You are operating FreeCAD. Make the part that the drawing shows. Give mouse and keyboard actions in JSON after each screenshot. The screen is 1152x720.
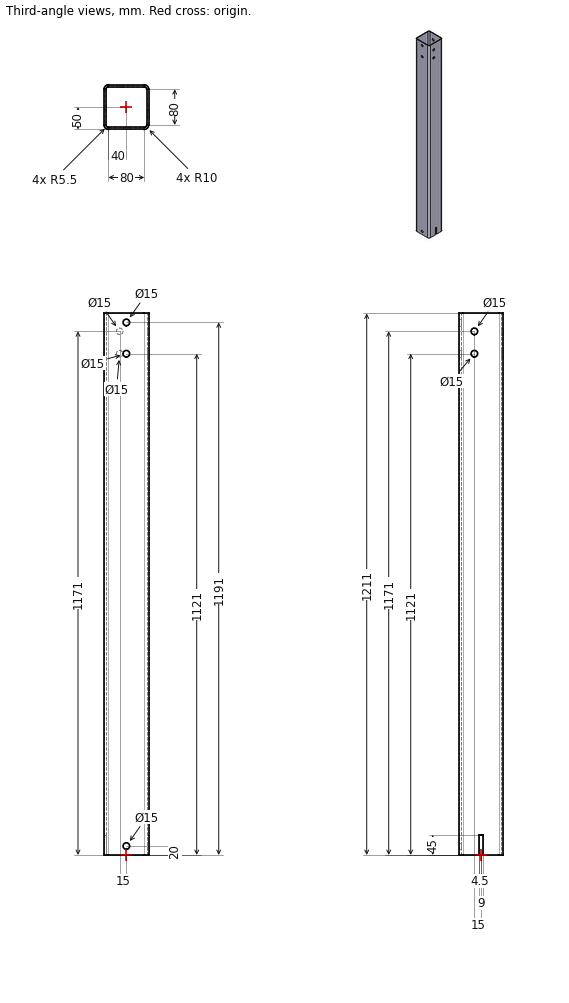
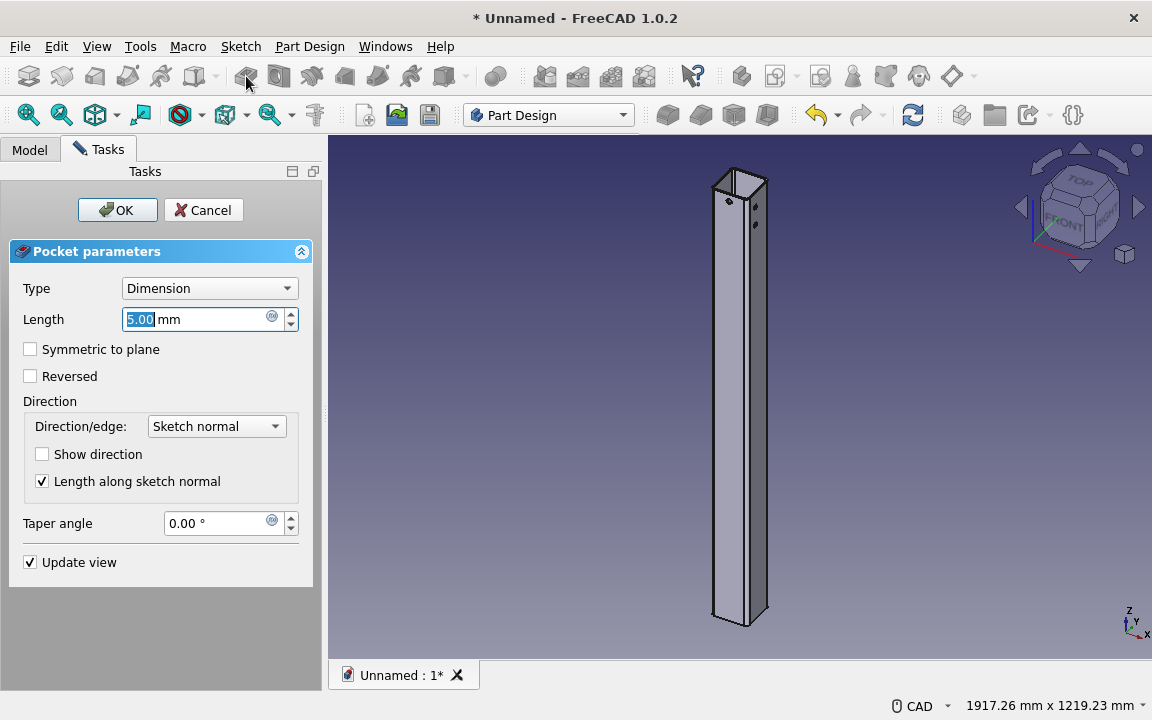
{"action": "left_click", "coordinate": [210, 288]}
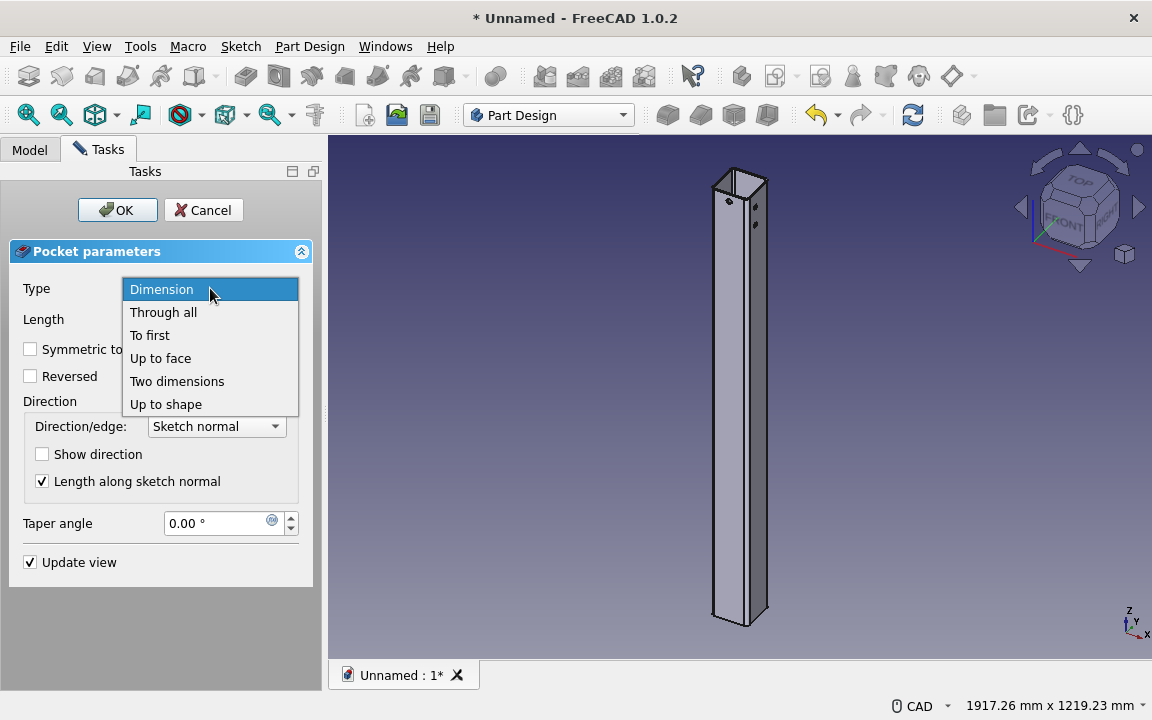
{"action": "left_click", "coordinate": [208, 336]}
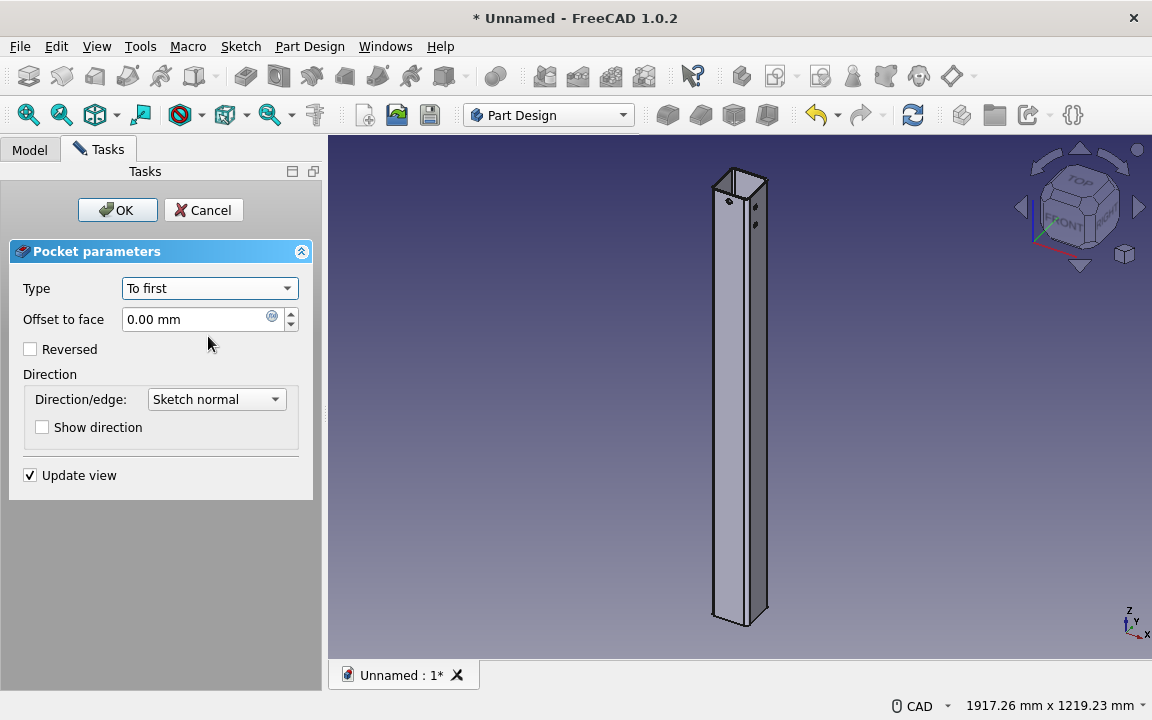
{"action": "left_click", "coordinate": [118, 210]}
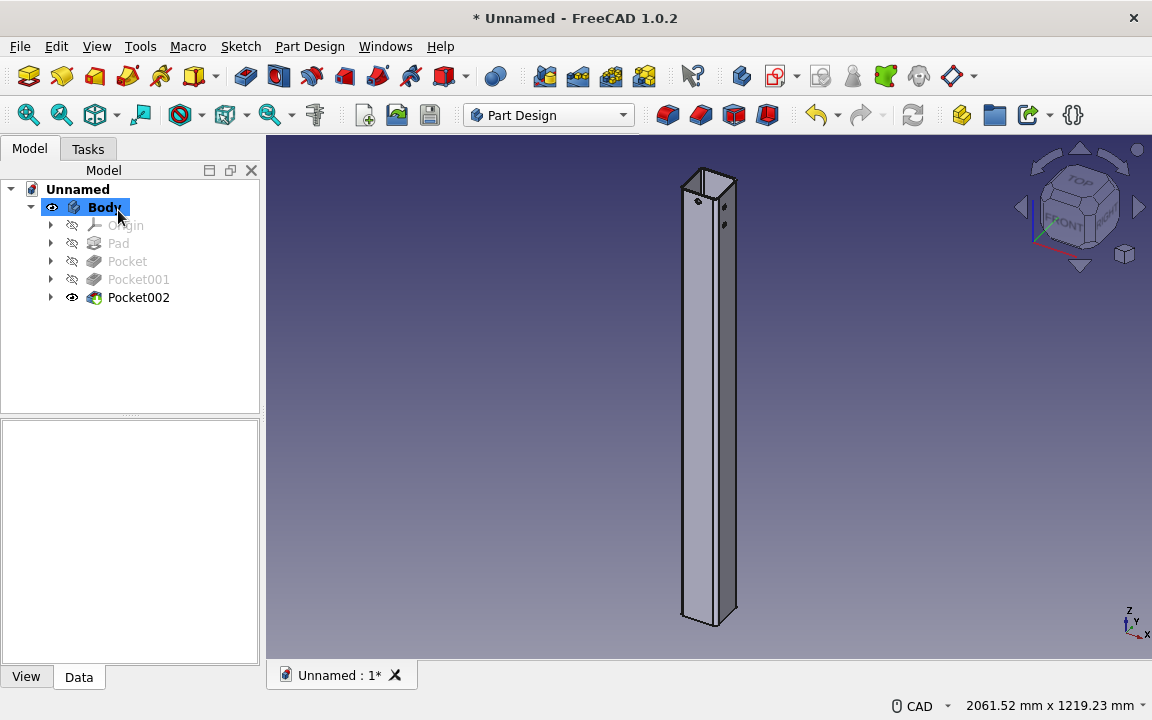
{"action": "left_click", "coordinate": [698, 224]}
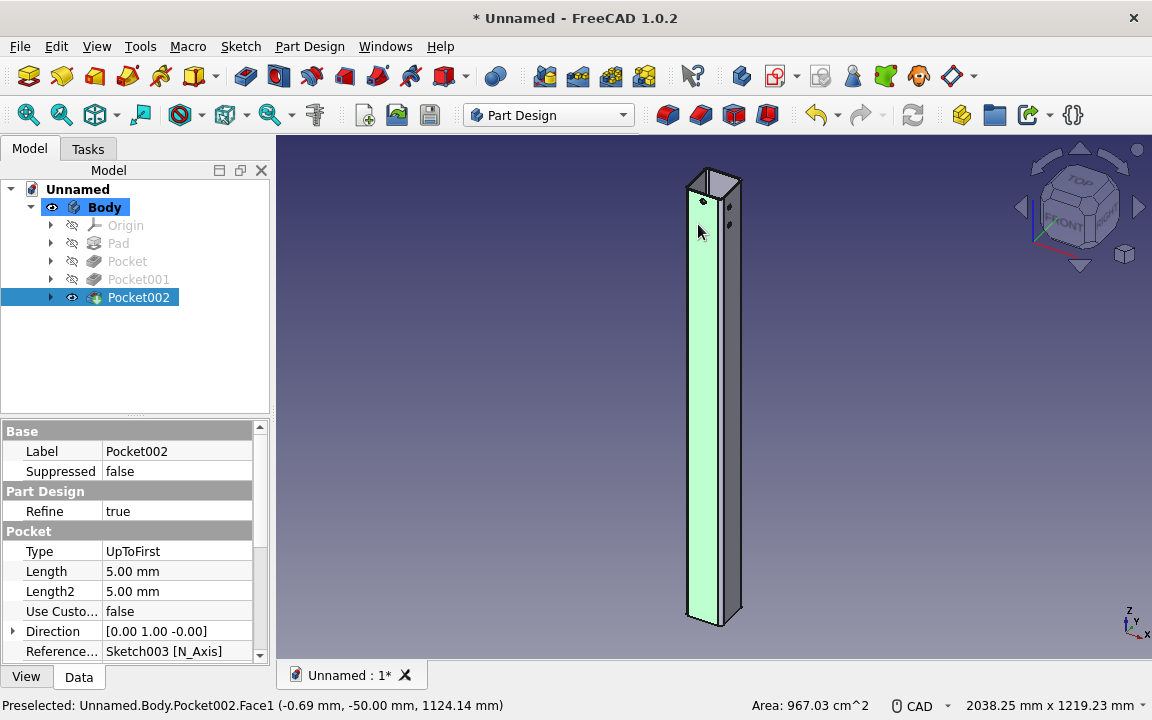
{"action": "left_click", "coordinate": [774, 76]}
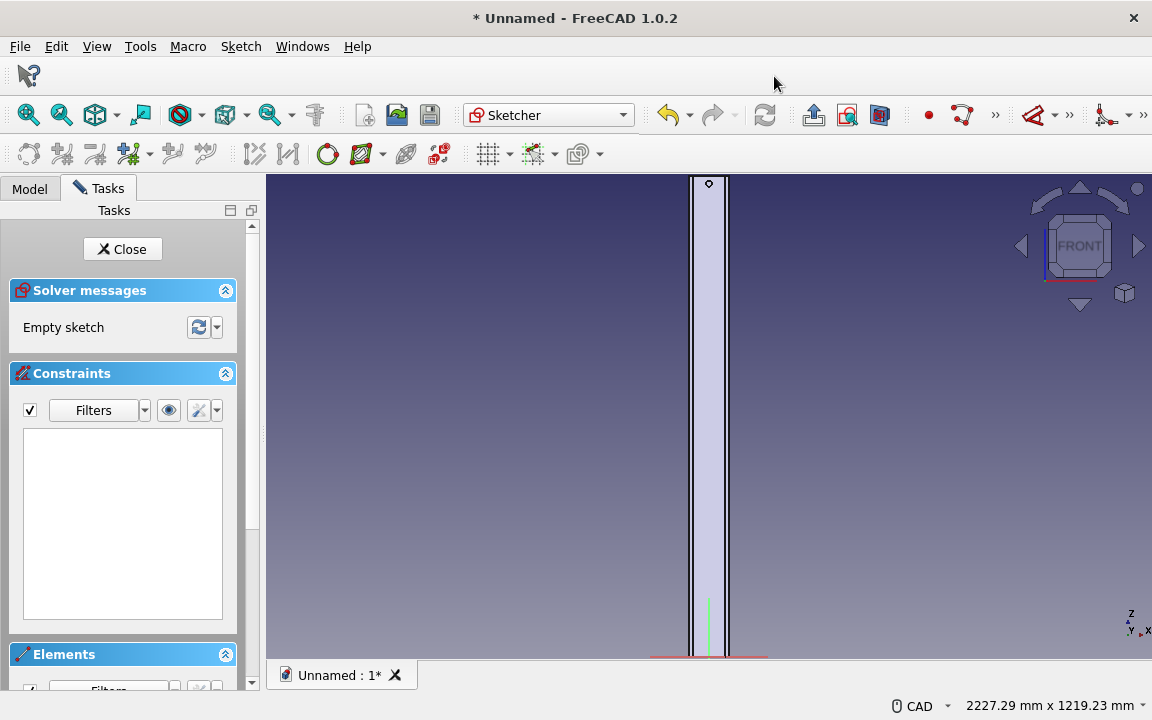
{"action": "scroll", "coordinate": [713, 202], "scroll_direction": "up", "scroll_amount": 15}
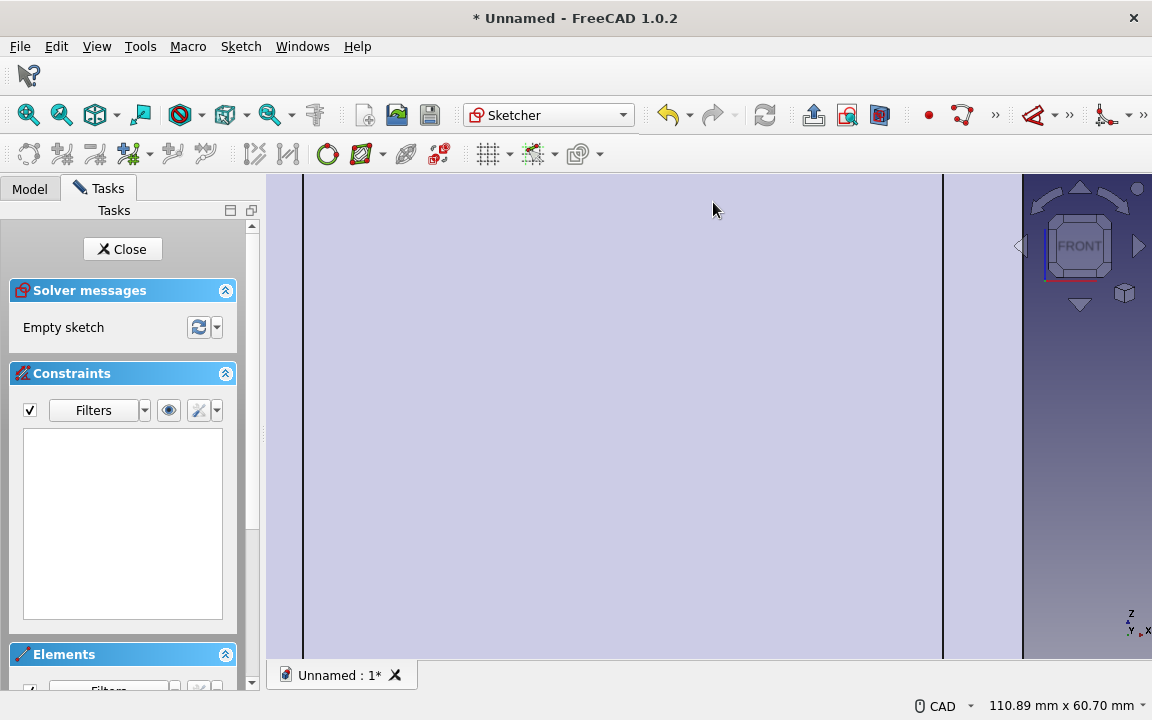
{"action": "scroll", "coordinate": [613, 375], "scroll_direction": "up", "scroll_amount": 5}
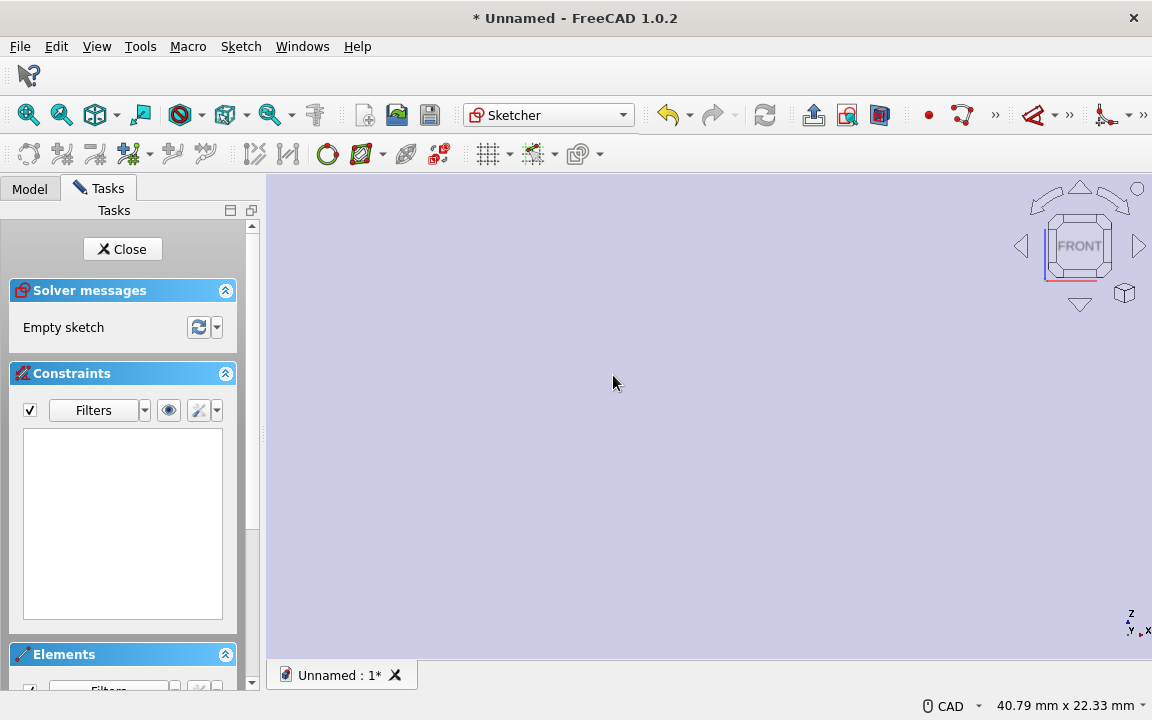
{"action": "key", "text": "g c"}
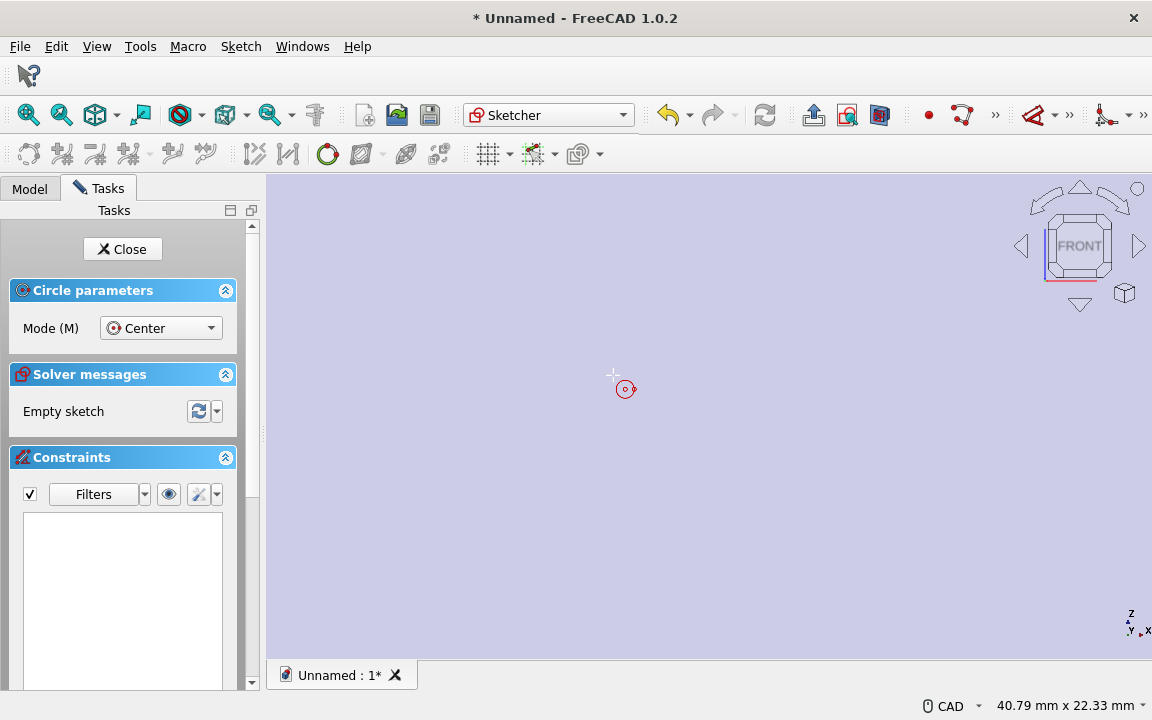
{"action": "left_click", "coordinate": [640, 416]}
{"action": "left_click", "coordinate": [755, 301]}
{"action": "key", "text": "Escape"}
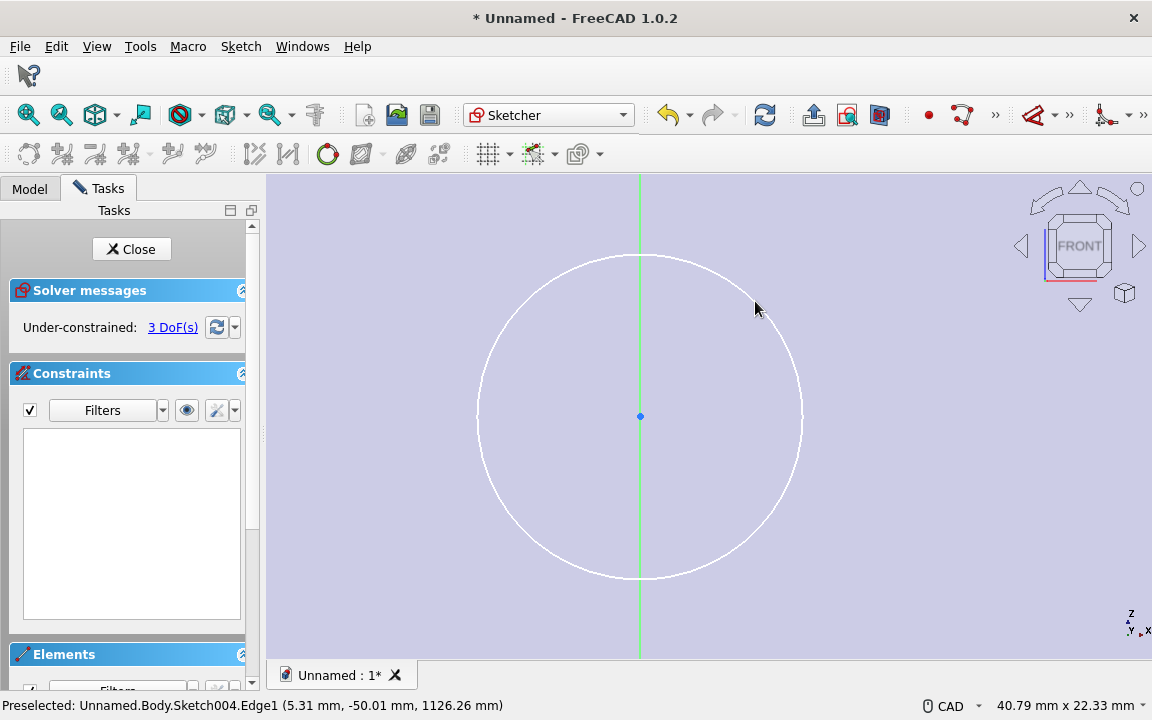
{"action": "left_click", "coordinate": [640, 417]}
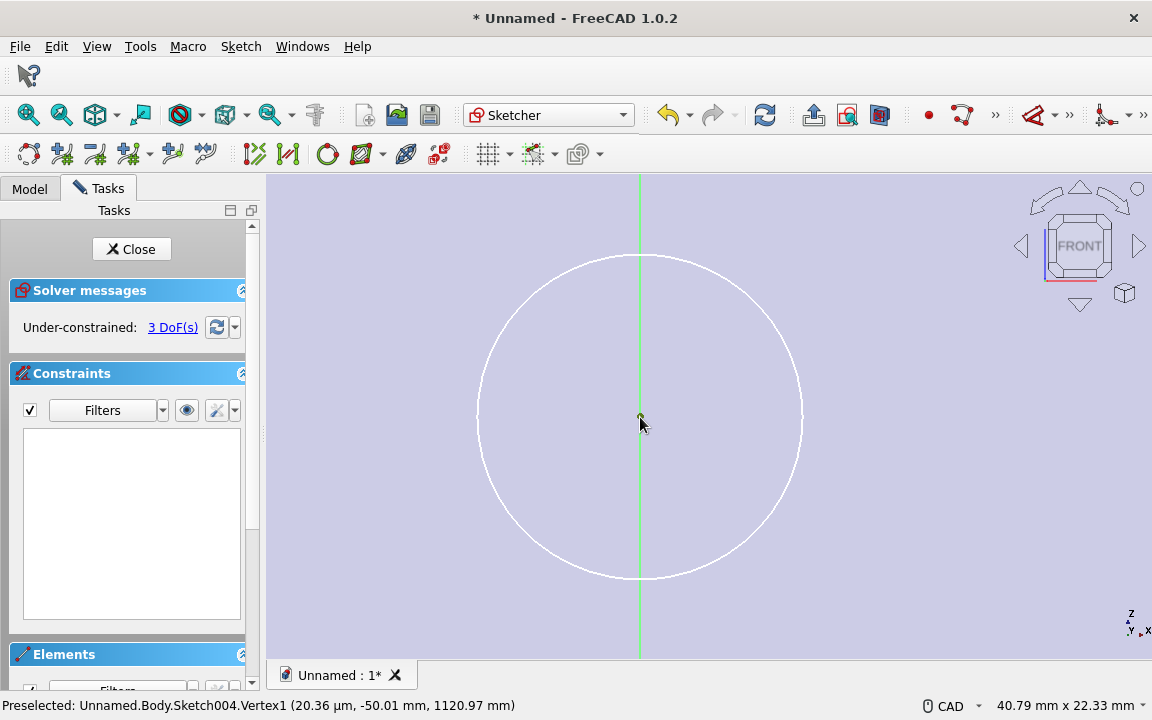
{"action": "left_click", "coordinate": [640, 539]}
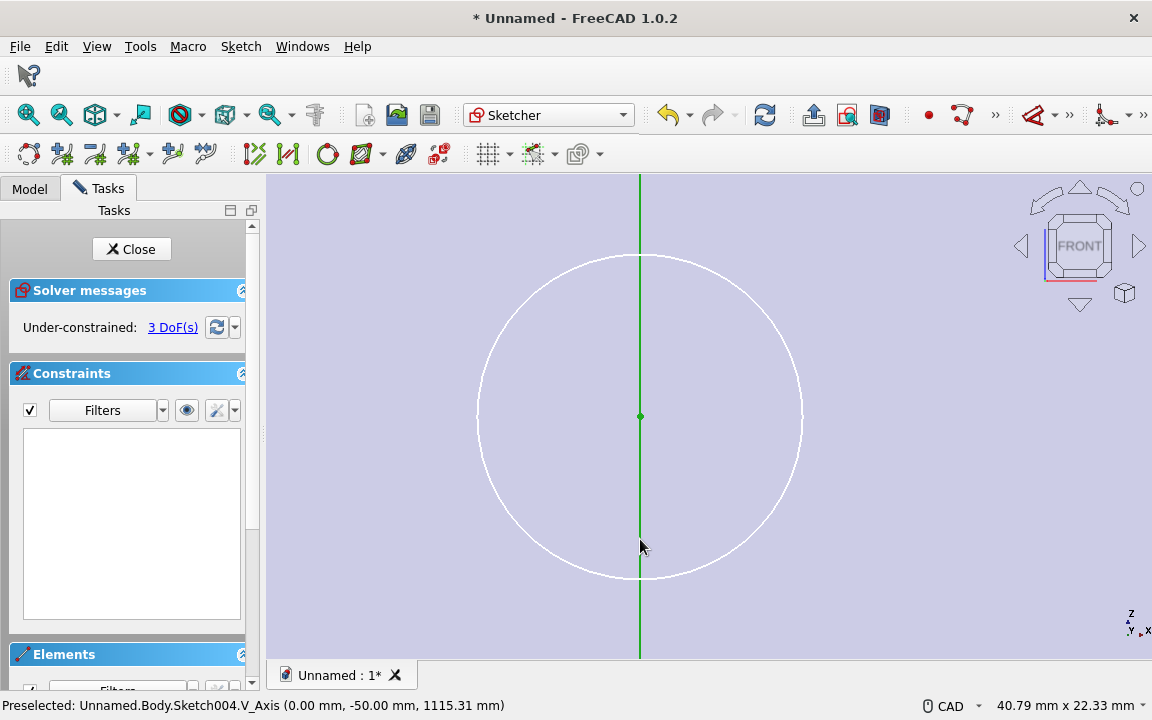
{"action": "key", "text": "c"}